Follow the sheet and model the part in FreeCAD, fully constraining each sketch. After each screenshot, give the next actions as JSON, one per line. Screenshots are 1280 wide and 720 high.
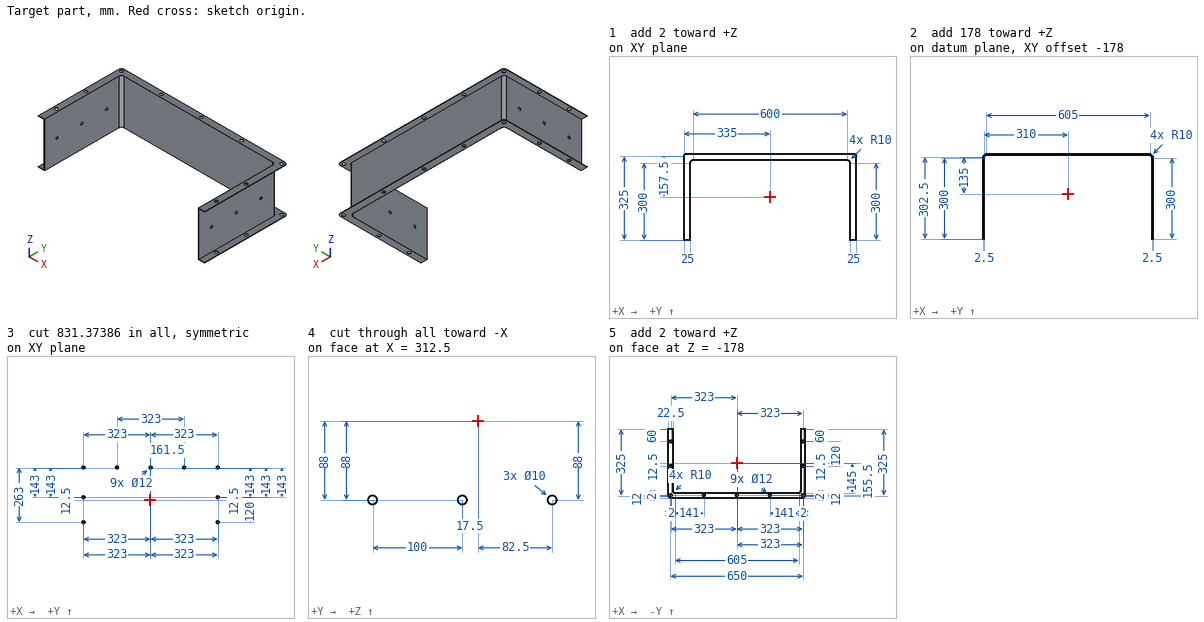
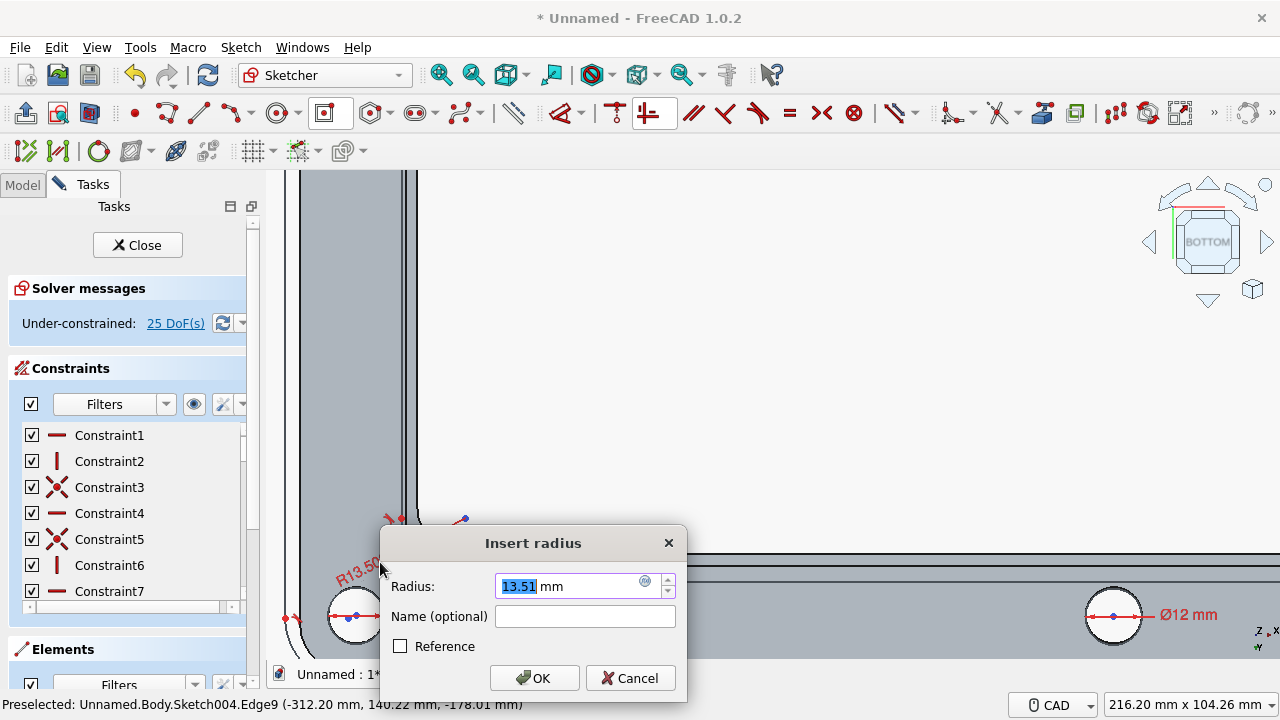
{"action": "type", "text": "10"}
{"action": "key", "text": "Return"}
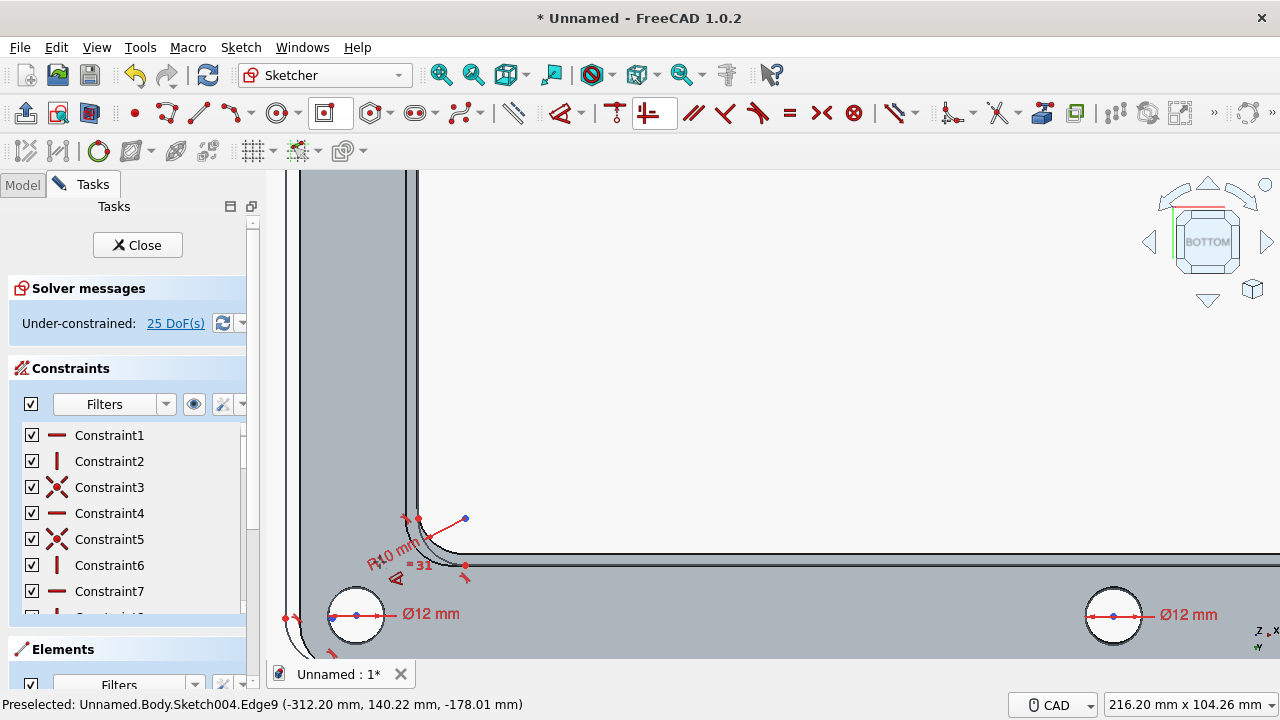
{"action": "scroll", "coordinate": [409, 548], "scroll_direction": "down", "scroll_amount": 8}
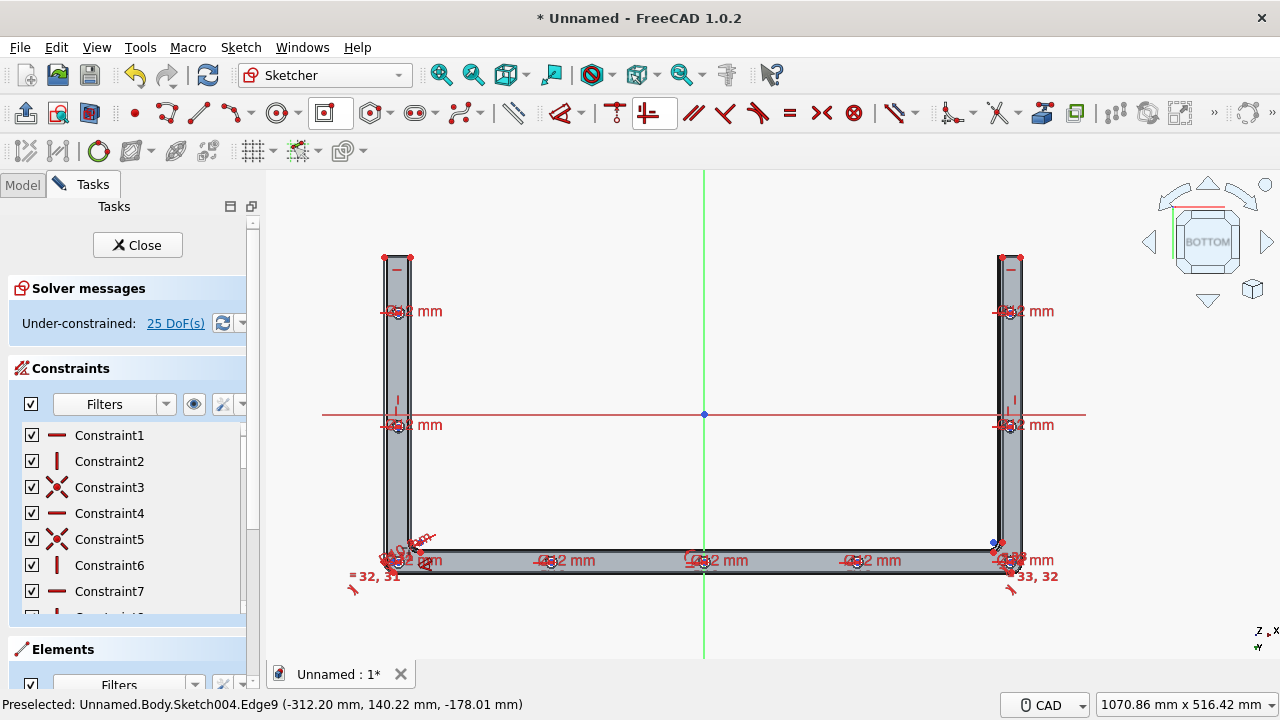
{"action": "scroll", "coordinate": [1011, 572], "scroll_direction": "up", "scroll_amount": 16}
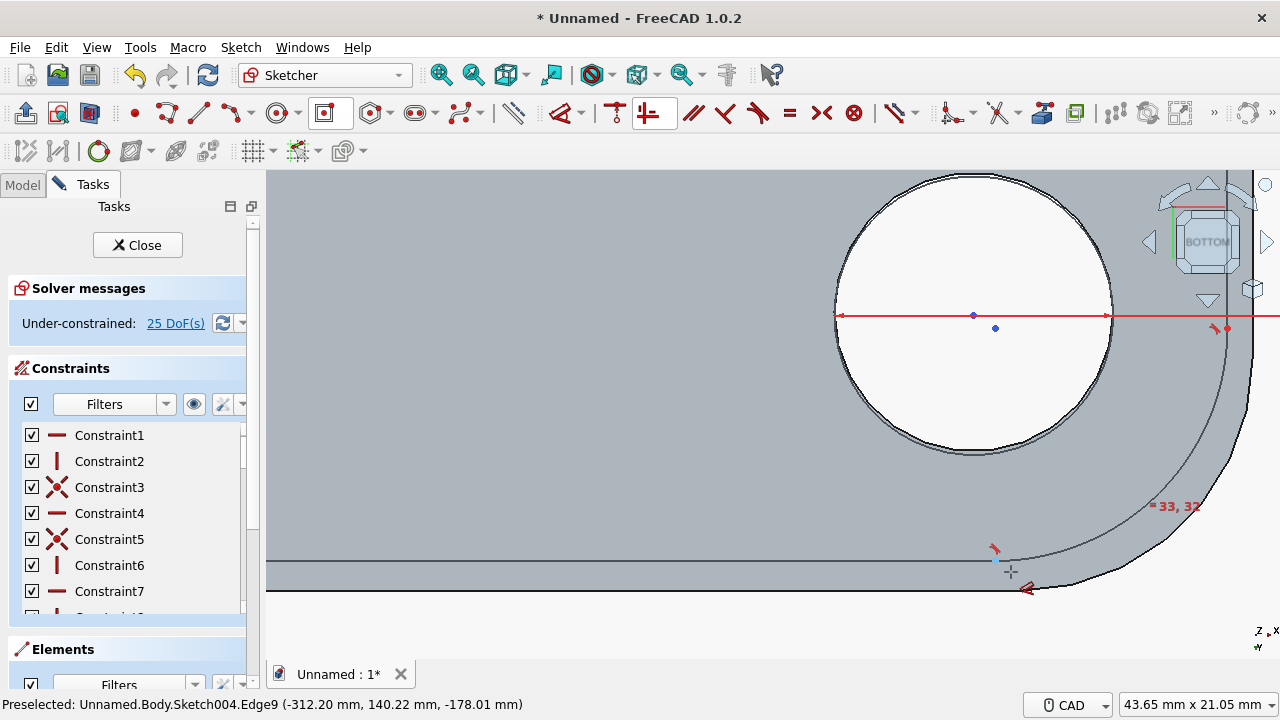
{"action": "left_click", "coordinate": [995, 561]}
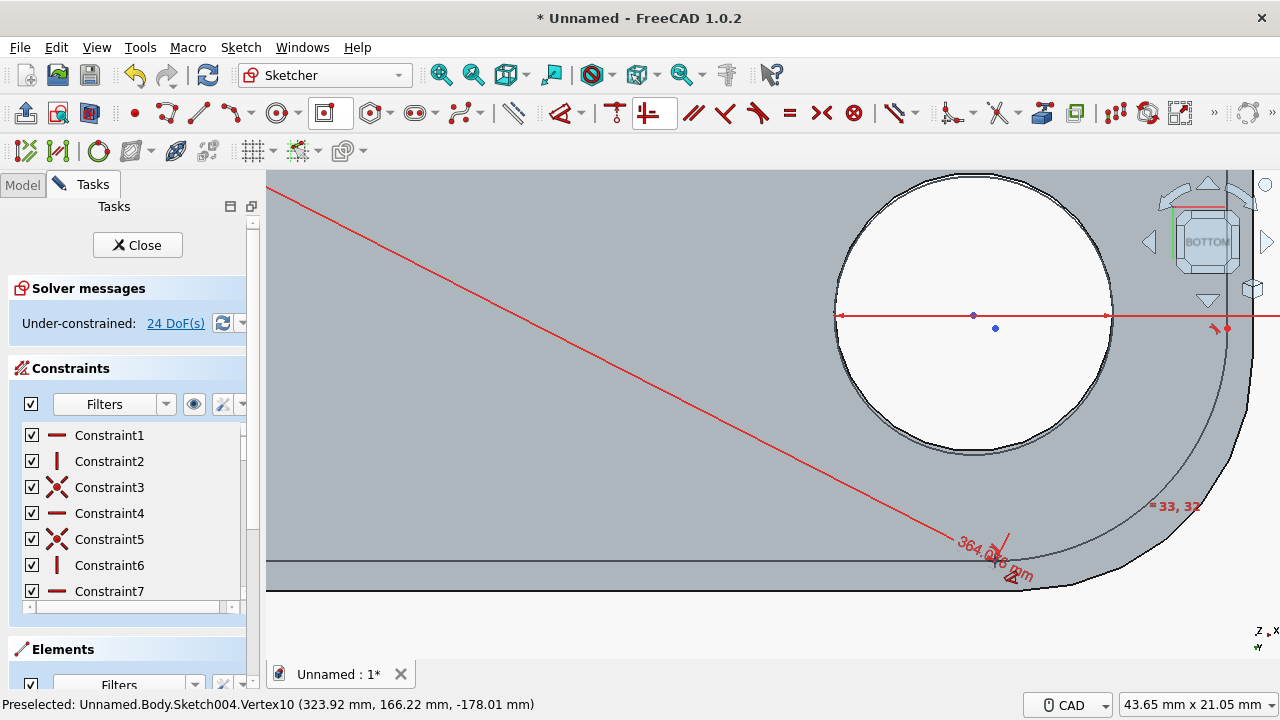
{"action": "left_click", "coordinate": [974, 316]}
{"action": "left_click", "coordinate": [984, 595]}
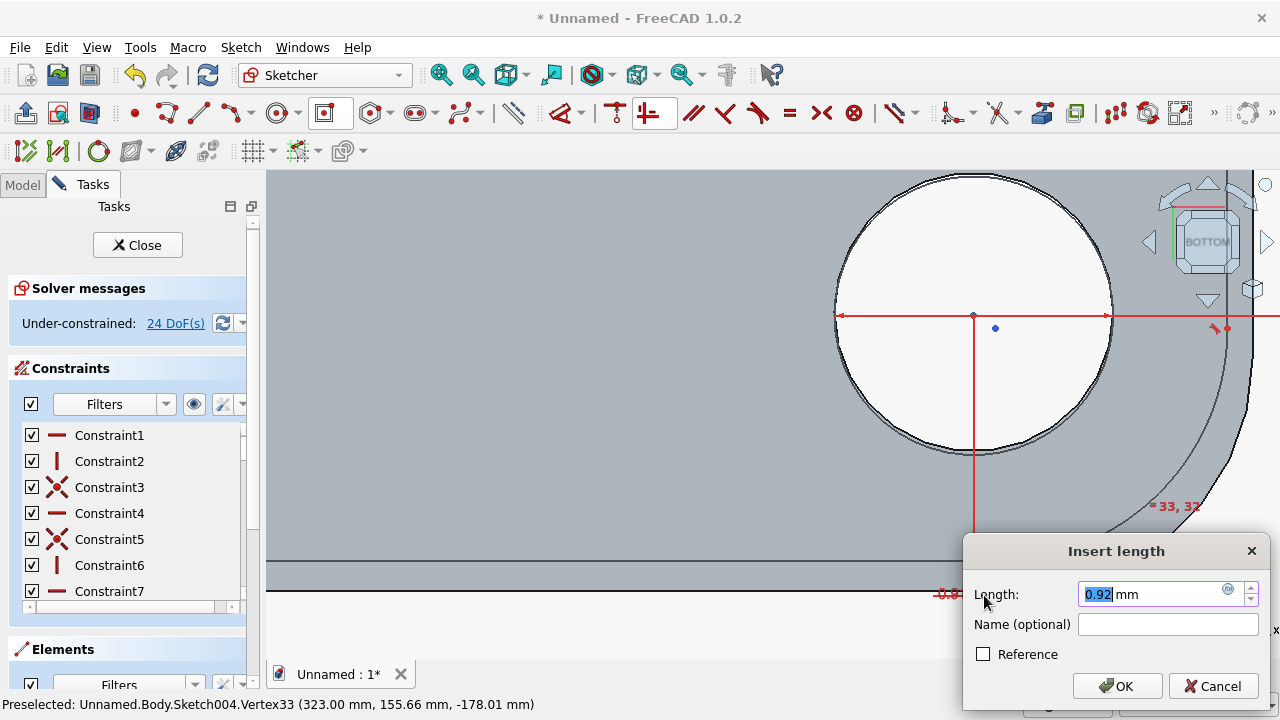
{"action": "type", "text": "2"}
{"action": "key", "text": "Return"}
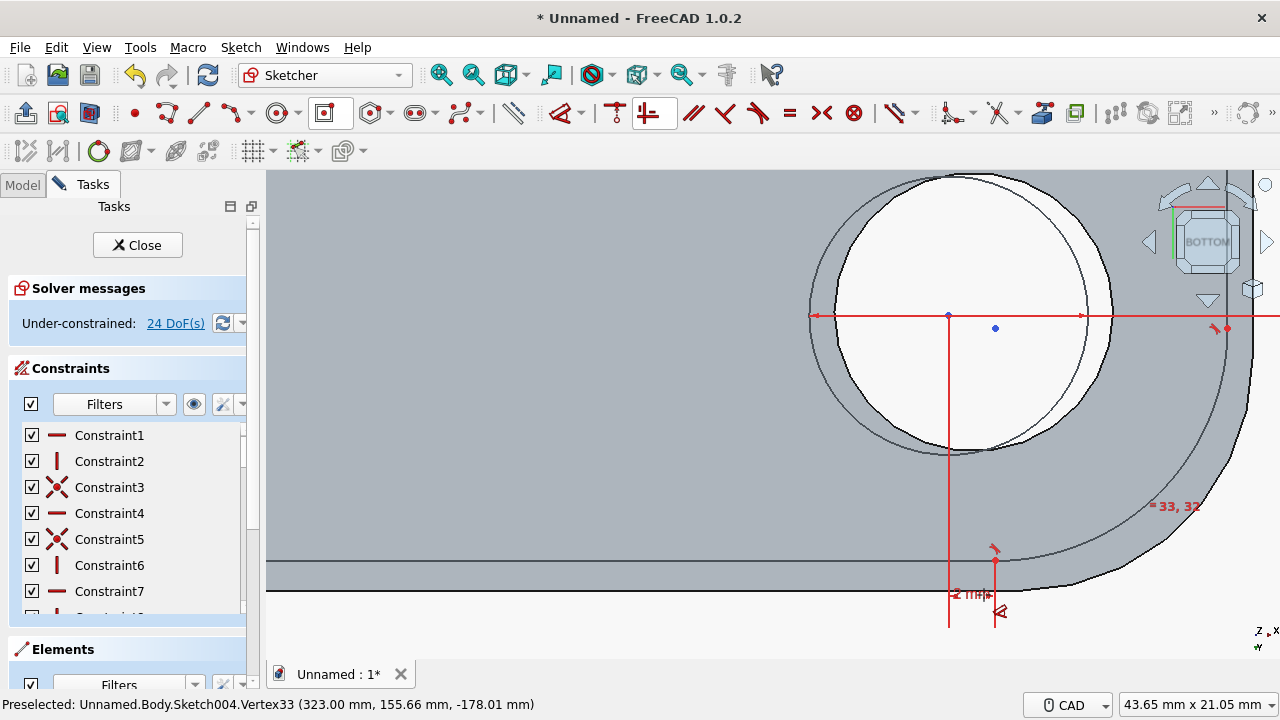
{"action": "scroll", "coordinate": [1012, 572], "scroll_direction": "down", "scroll_amount": 16}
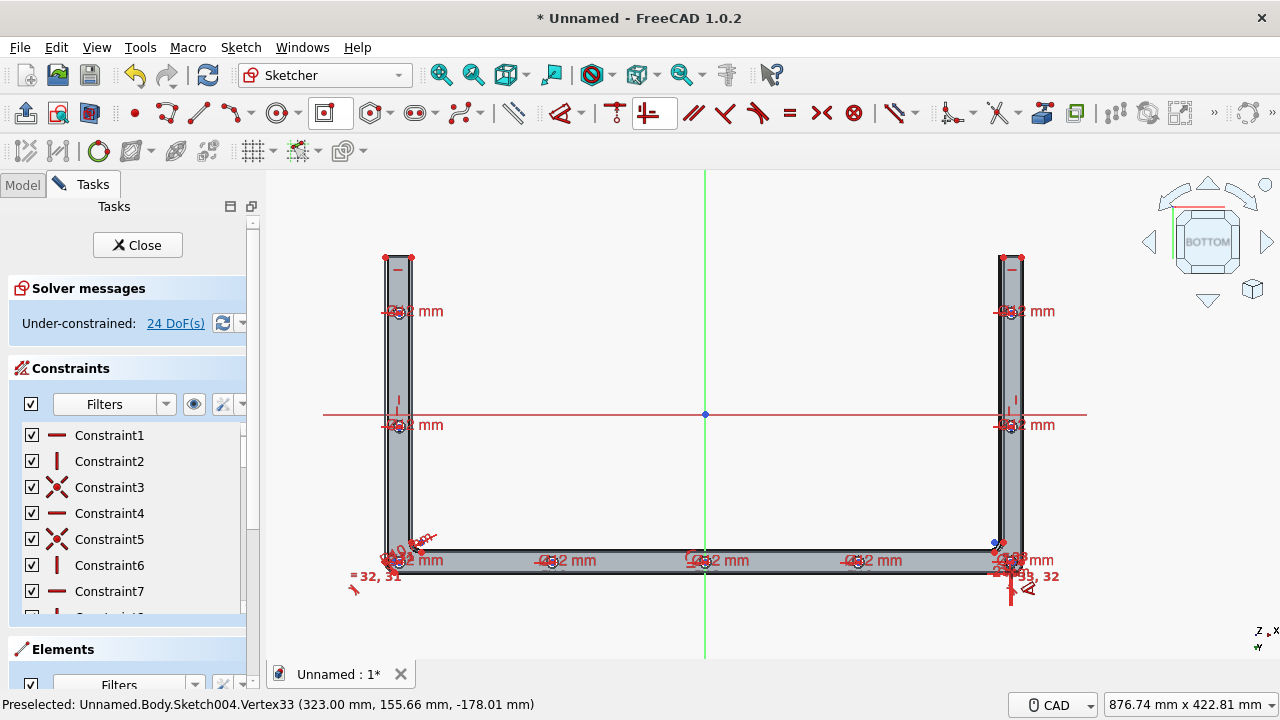
{"action": "scroll", "coordinate": [1021, 563], "scroll_direction": "up", "scroll_amount": 16}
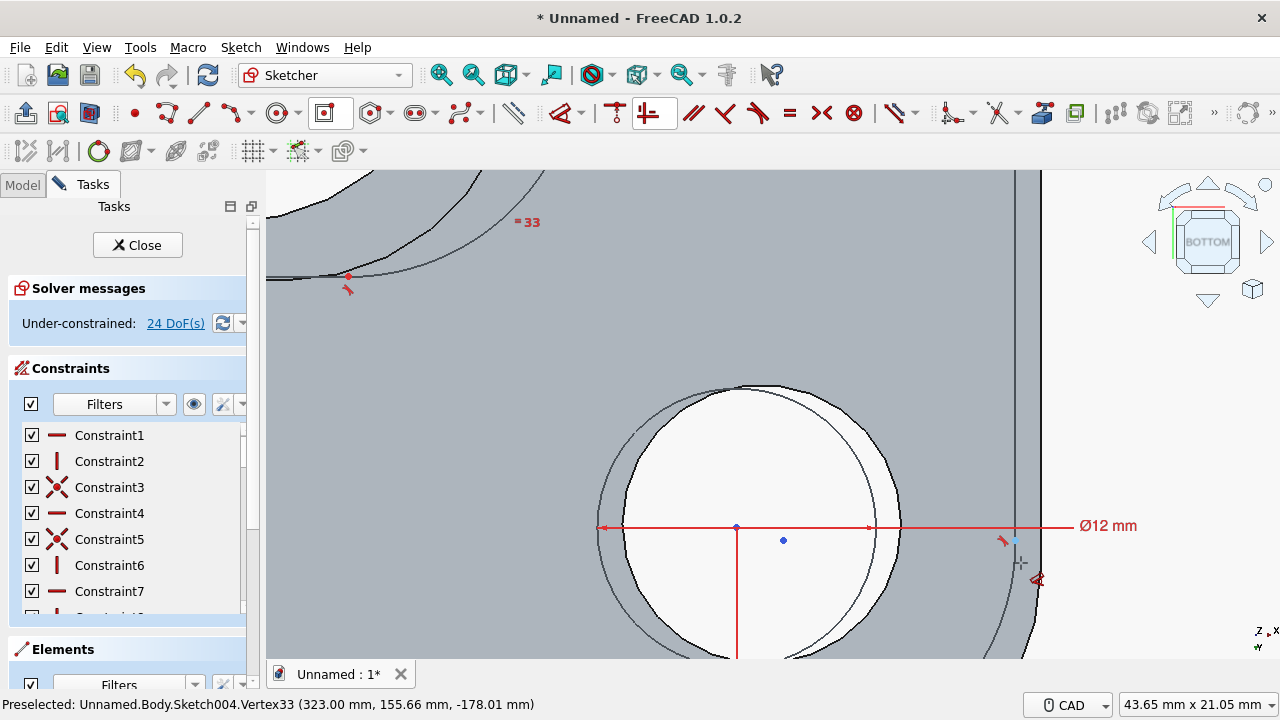
{"action": "left_click", "coordinate": [1015, 541]}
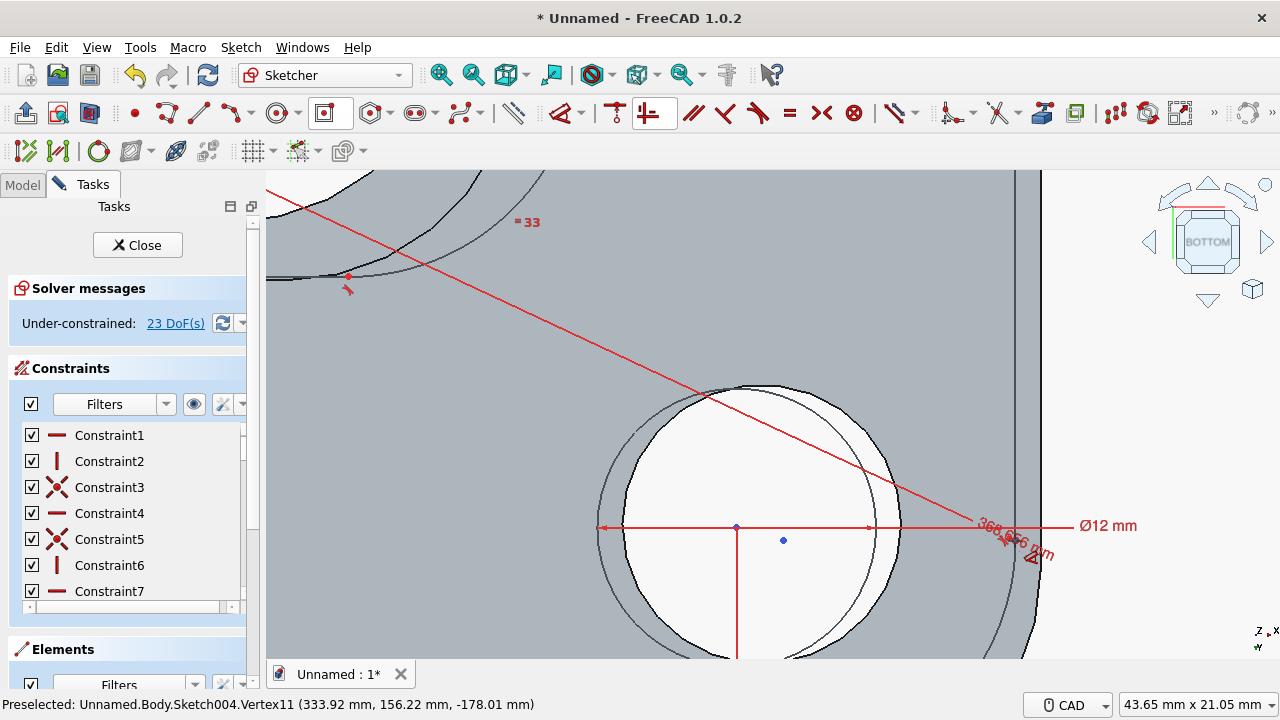
{"action": "left_click", "coordinate": [737, 528]}
{"action": "left_click", "coordinate": [1049, 534]}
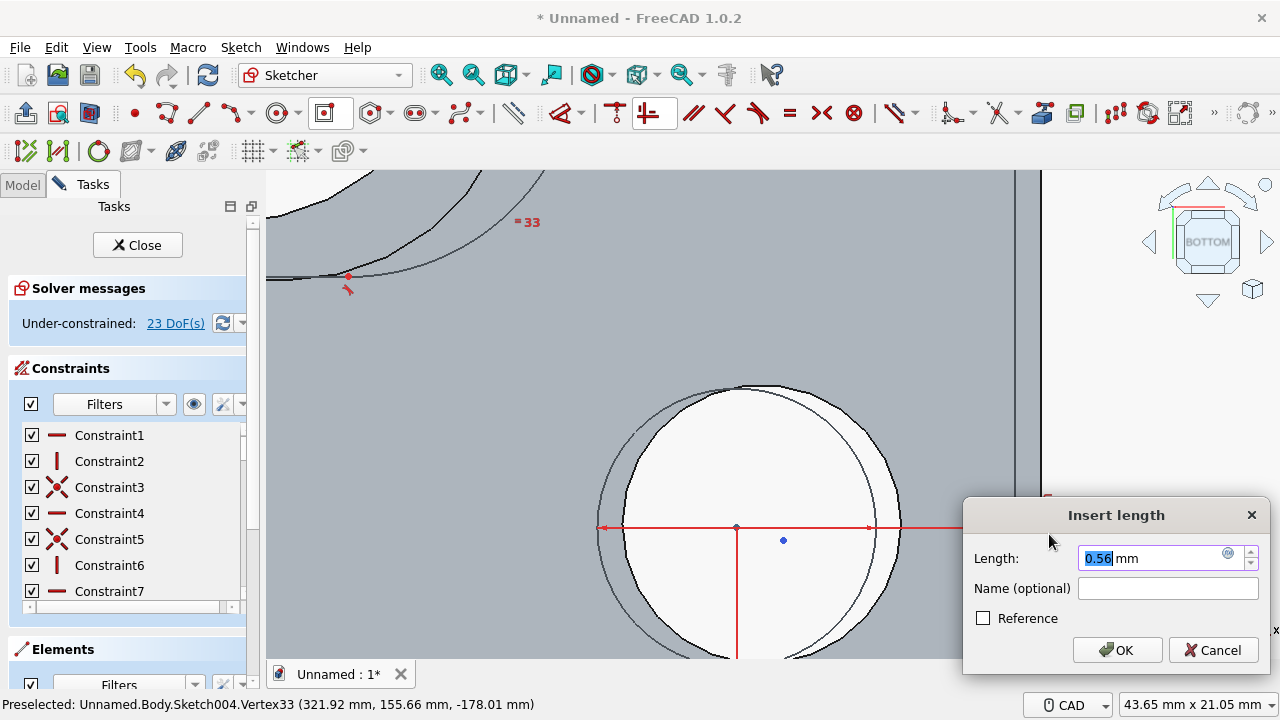
{"action": "type", "text": "2"}
{"action": "key", "text": "Return"}